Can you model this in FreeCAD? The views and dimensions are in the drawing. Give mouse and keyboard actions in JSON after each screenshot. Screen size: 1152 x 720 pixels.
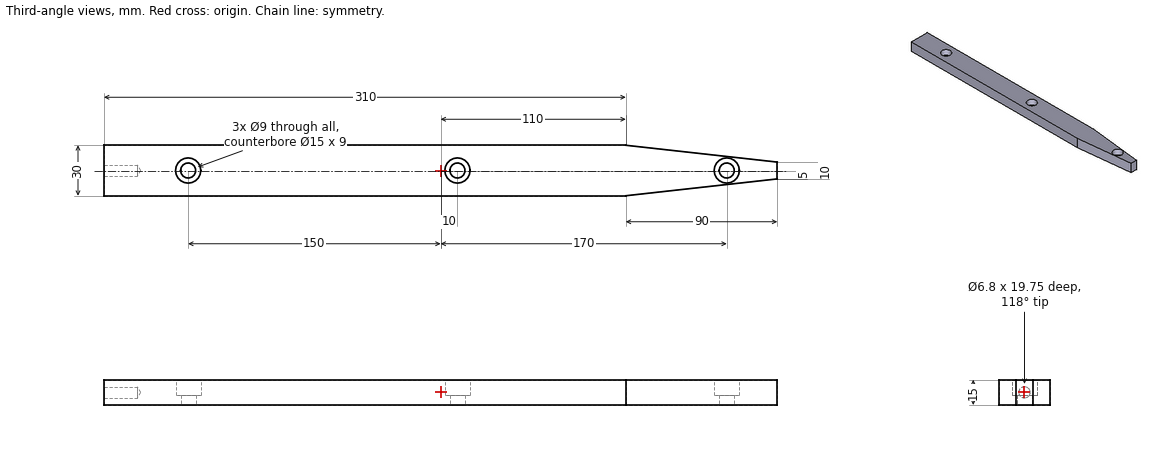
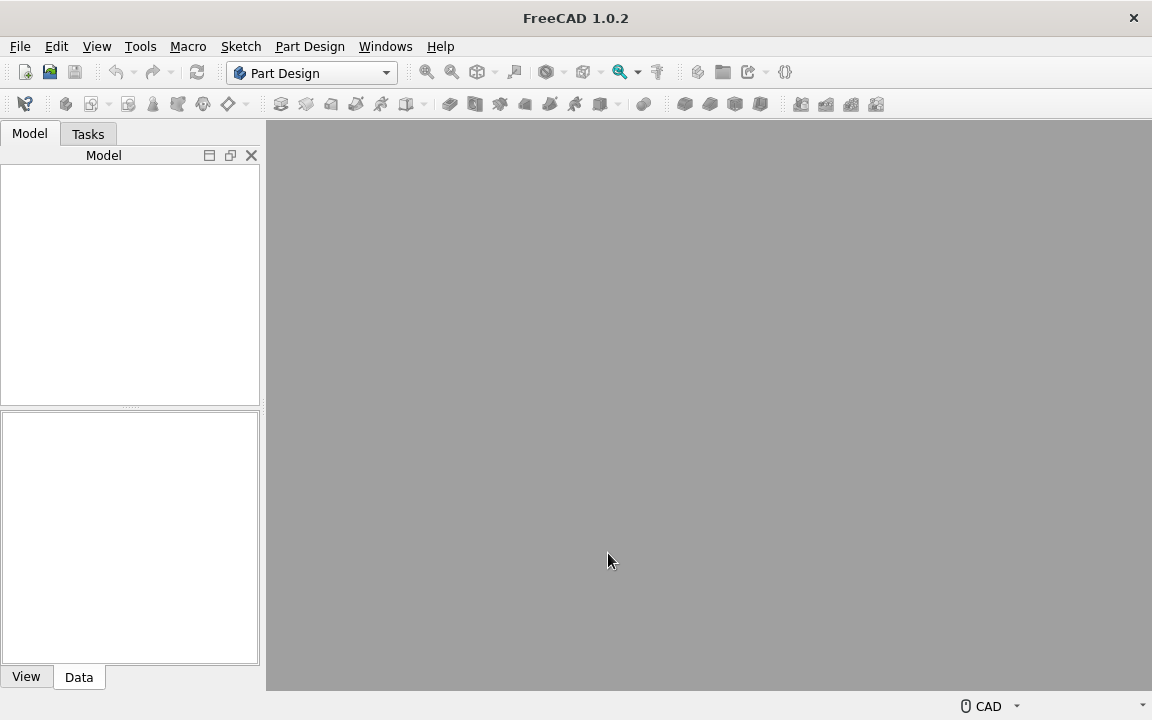
{"action": "key", "text": "ctrl+n"}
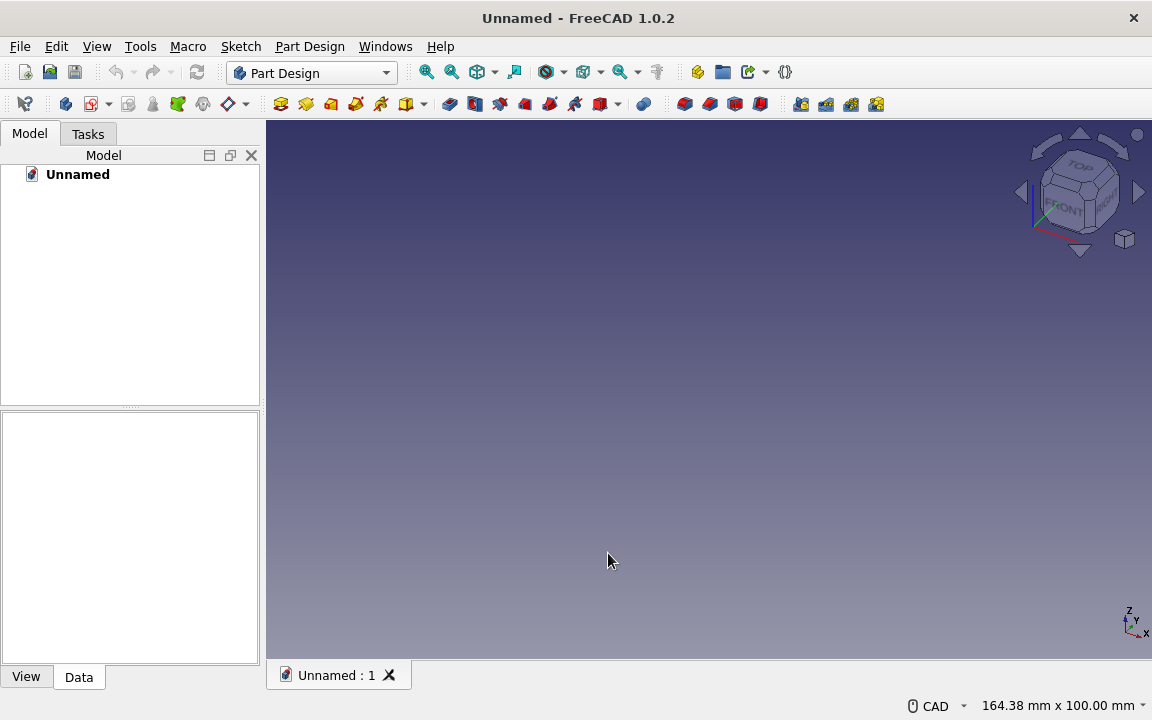
{"action": "left_click", "coordinate": [90, 104]}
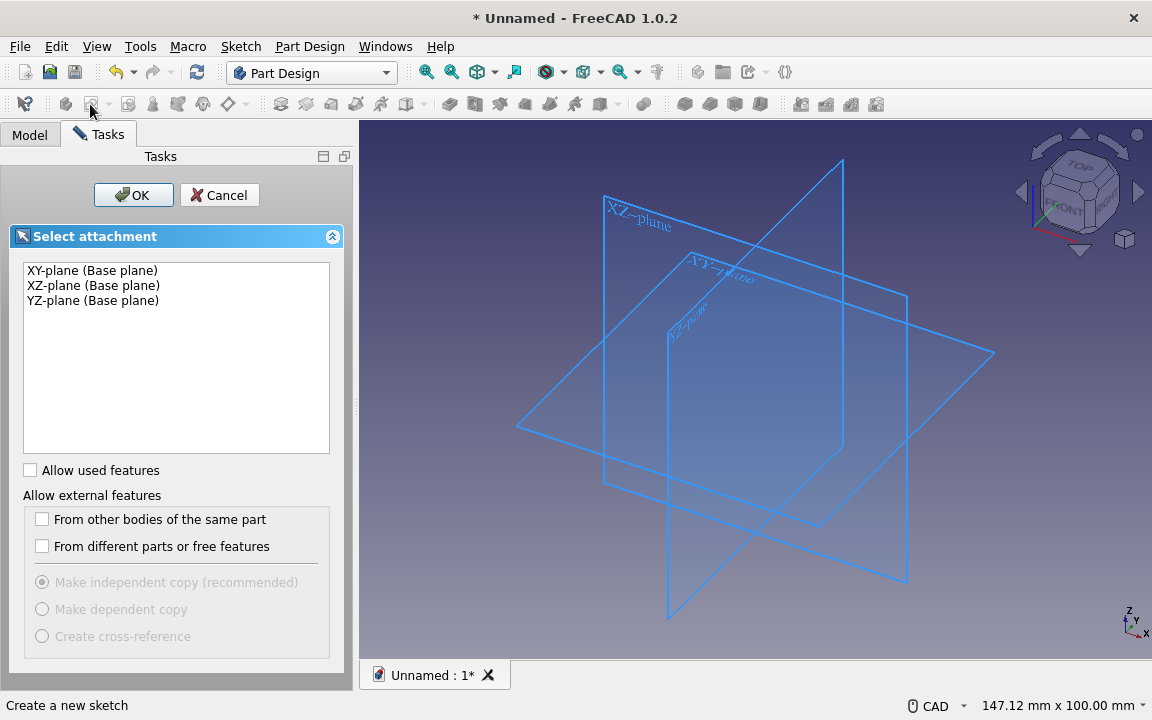
{"action": "left_click", "coordinate": [84, 270]}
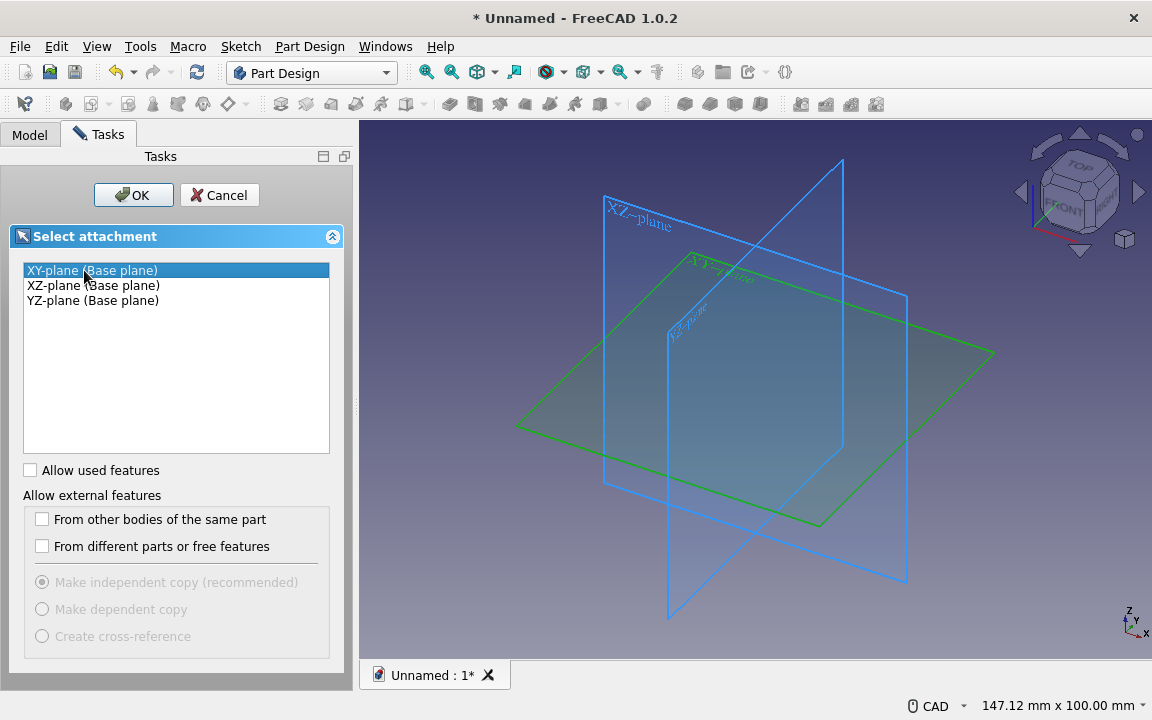
{"action": "left_click", "coordinate": [134, 195]}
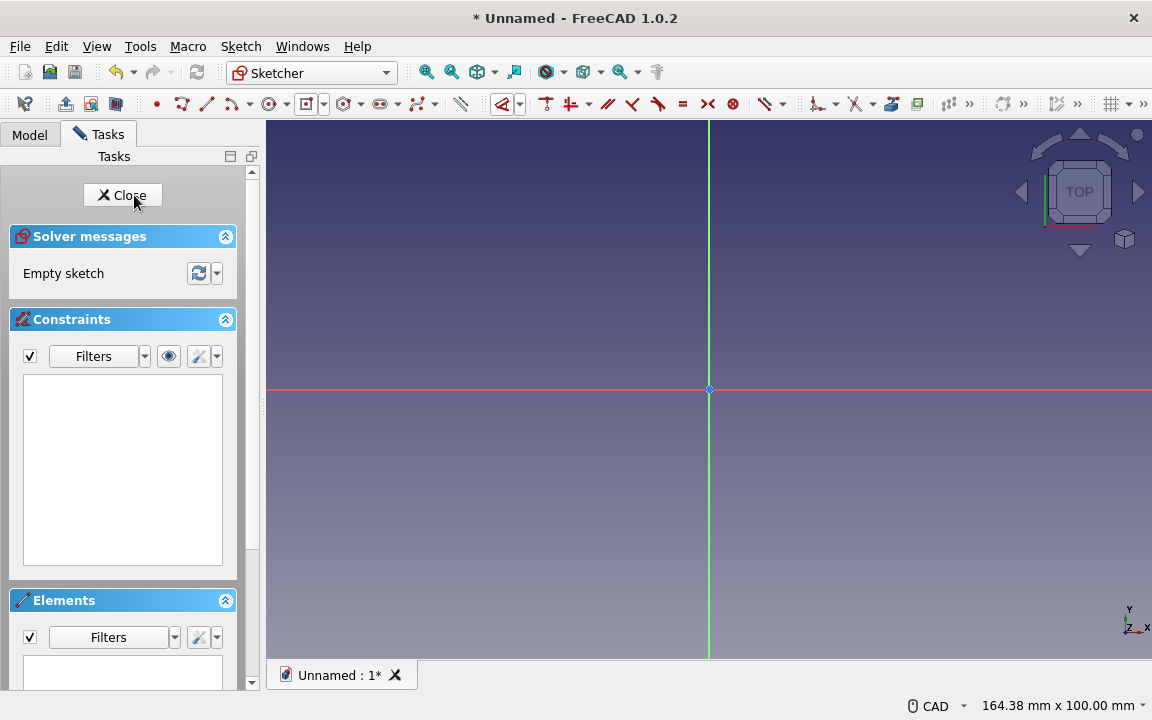
{"action": "scroll", "coordinate": [618, 390], "scroll_direction": "down", "scroll_amount": 7}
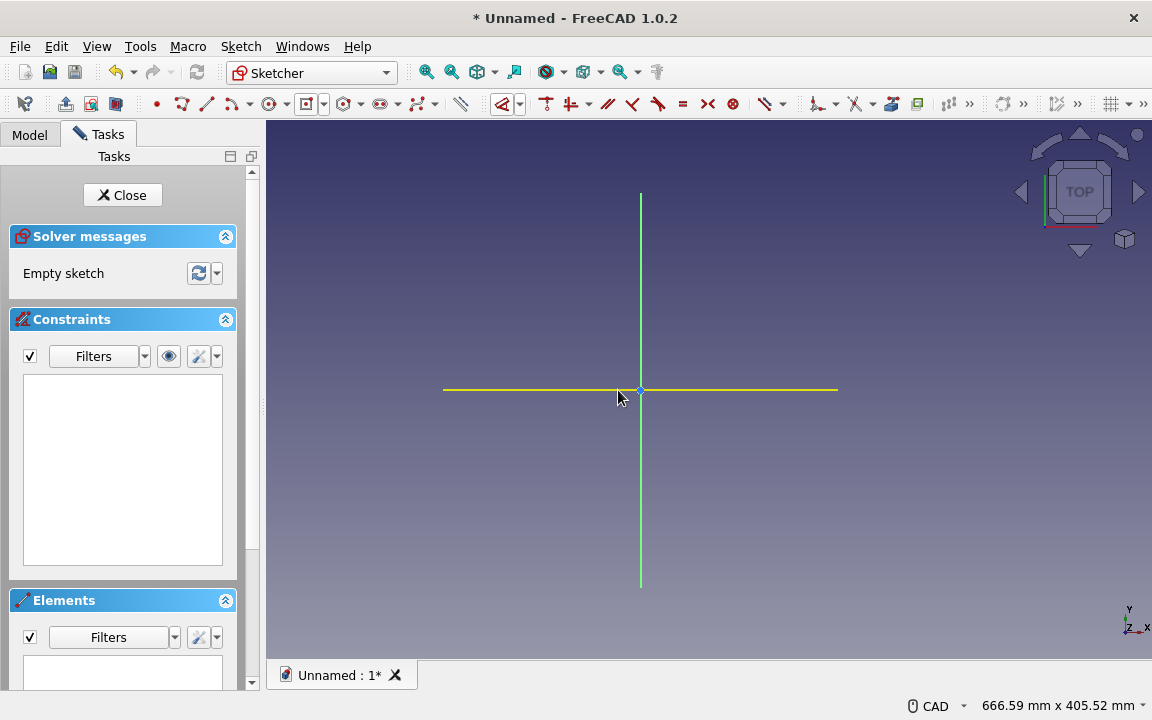
{"action": "key", "text": "g m"}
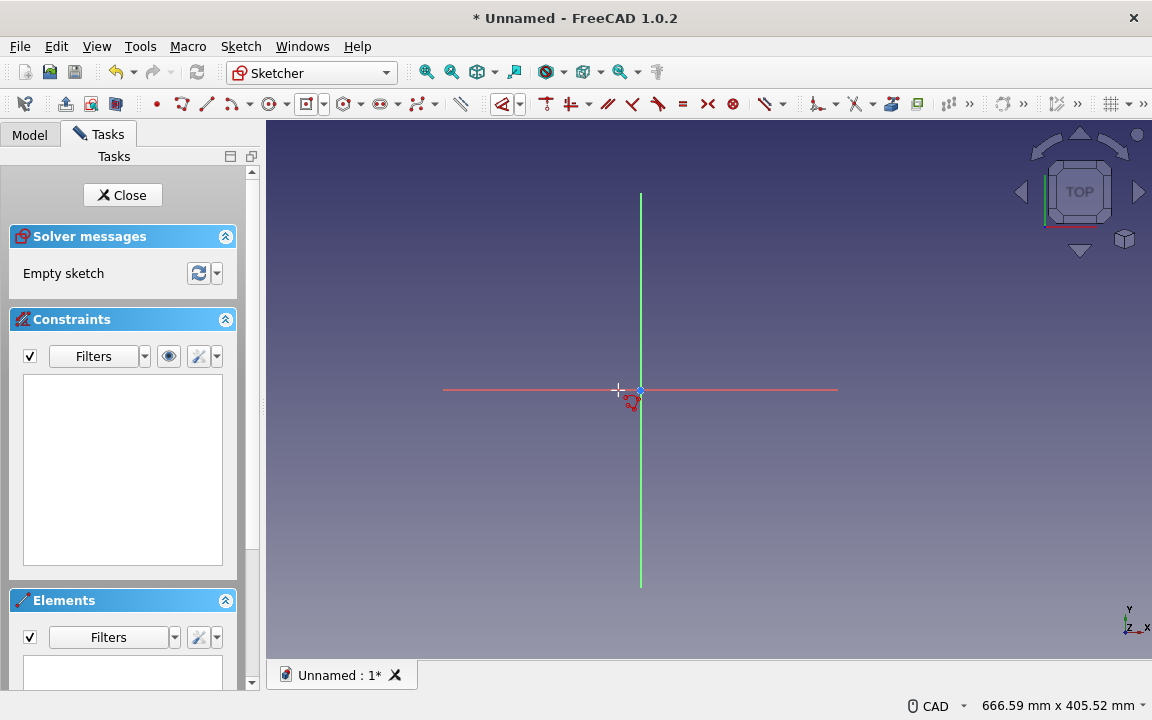
{"action": "left_click", "coordinate": [787, 370]}
{"action": "left_click", "coordinate": [375, 370]}
{"action": "left_click", "coordinate": [375, 410]}
{"action": "left_click", "coordinate": [787, 410]}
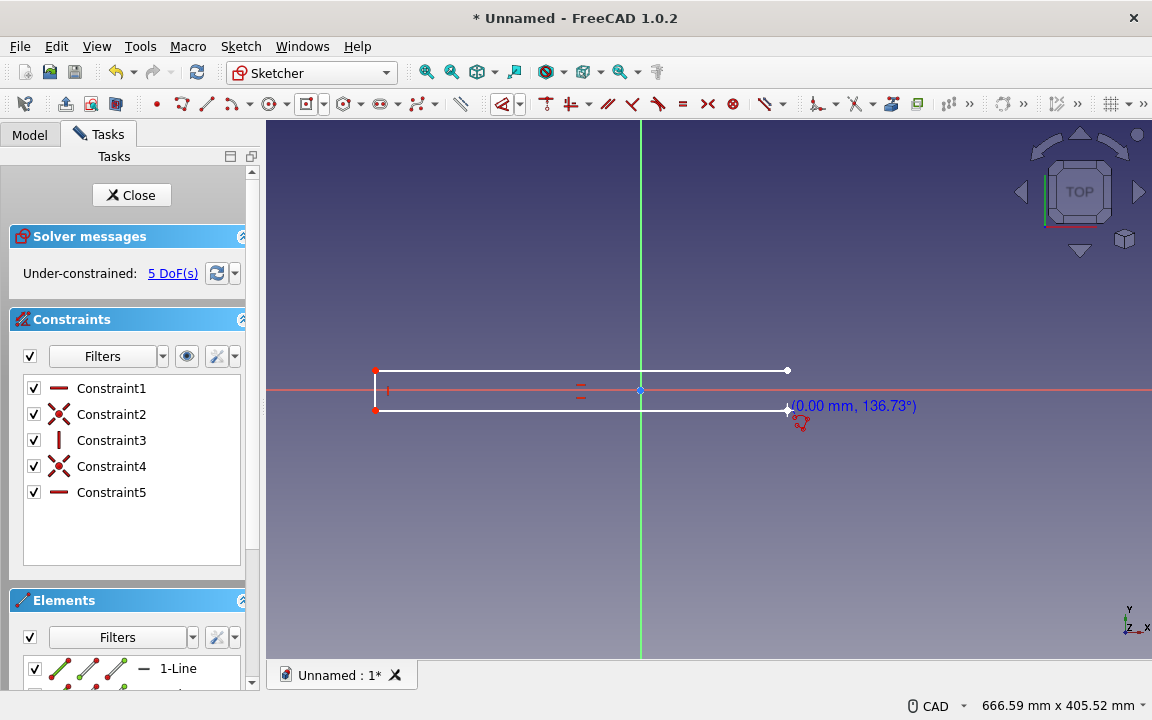
{"action": "scroll", "coordinate": [907, 397], "scroll_direction": "up", "scroll_amount": 5}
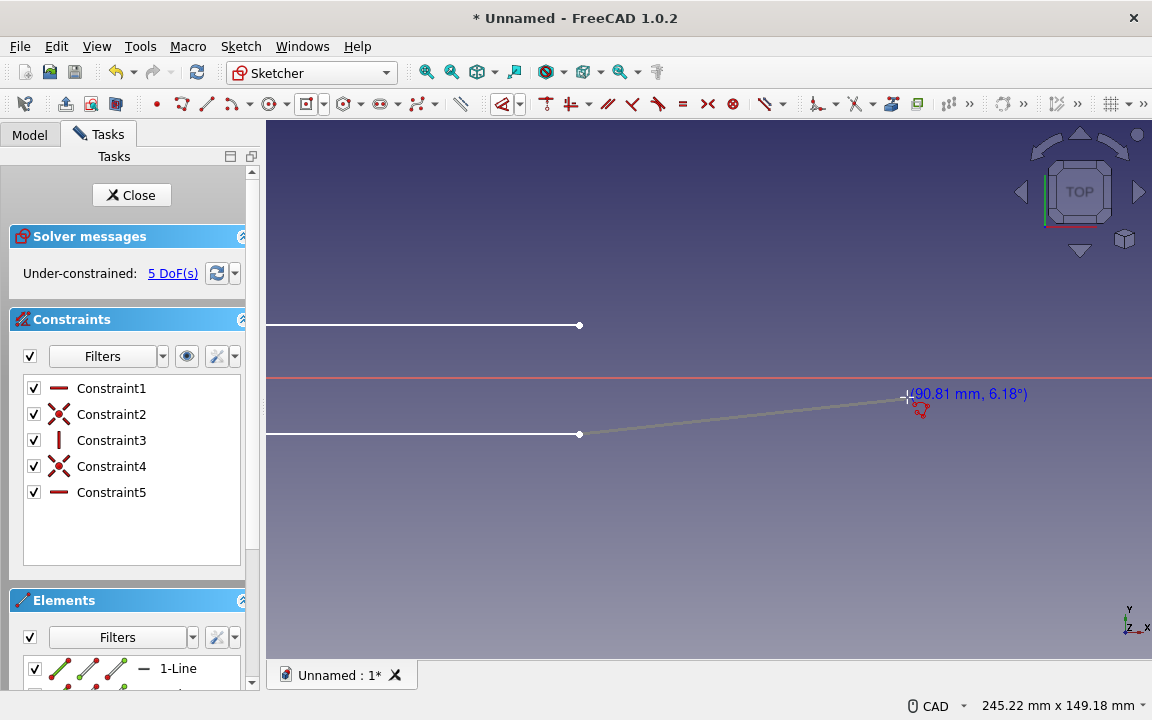
{"action": "left_click", "coordinate": [905, 396]}
{"action": "left_click", "coordinate": [905, 360]}
{"action": "left_click", "coordinate": [580, 325]}
{"action": "key", "text": "Escape"}
{"action": "key", "text": "Escape"}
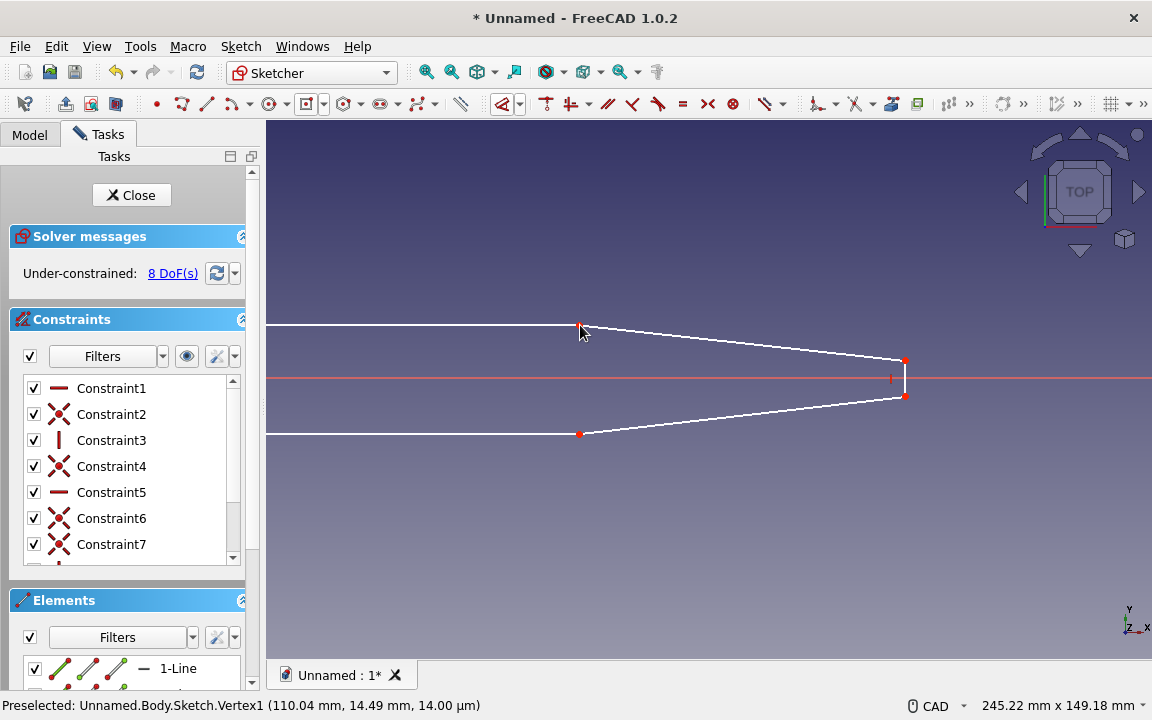
{"action": "left_click", "coordinate": [580, 325]}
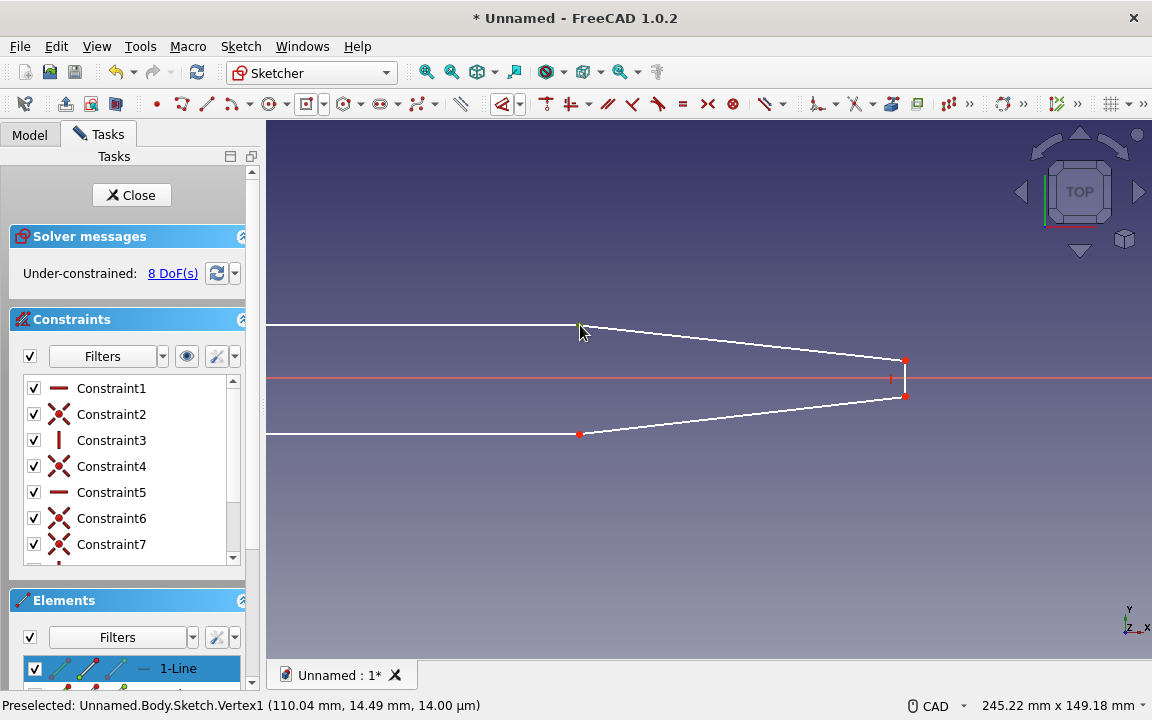
{"action": "left_click", "coordinate": [580, 434]}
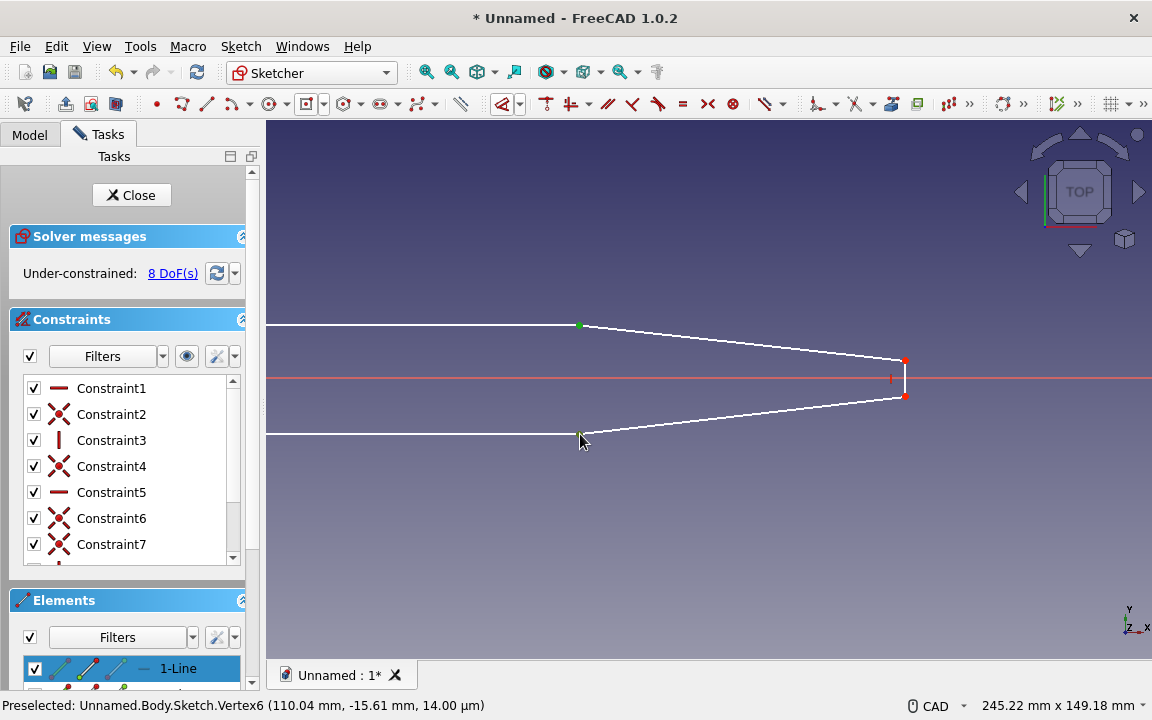
{"action": "left_click", "coordinate": [344, 378]}